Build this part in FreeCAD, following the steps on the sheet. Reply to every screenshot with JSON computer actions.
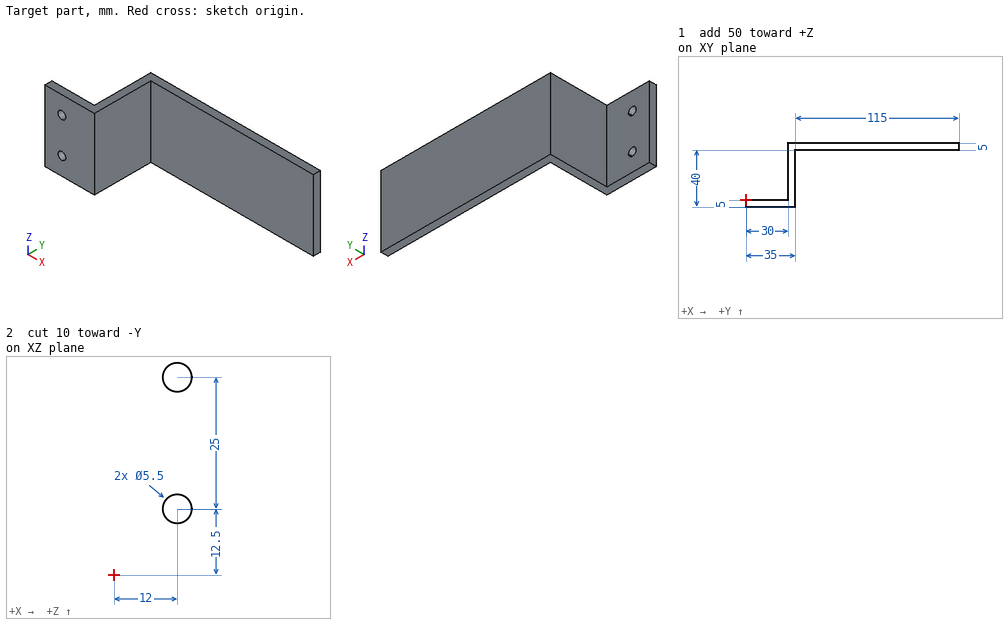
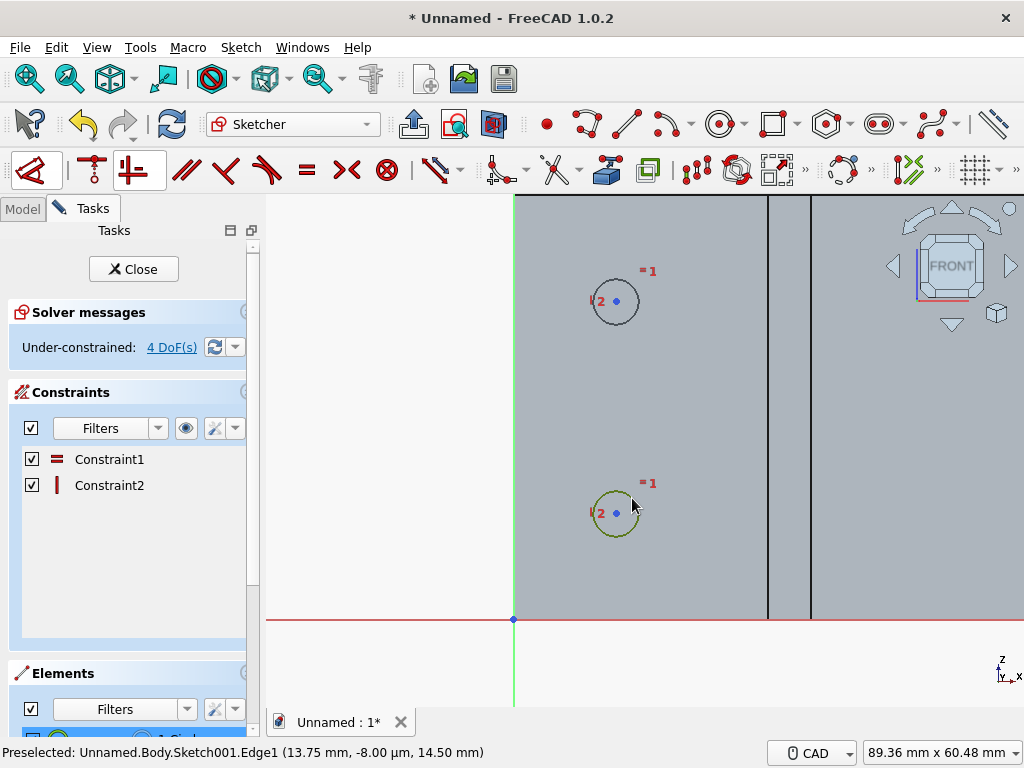
{"action": "left_click", "coordinate": [56, 170]}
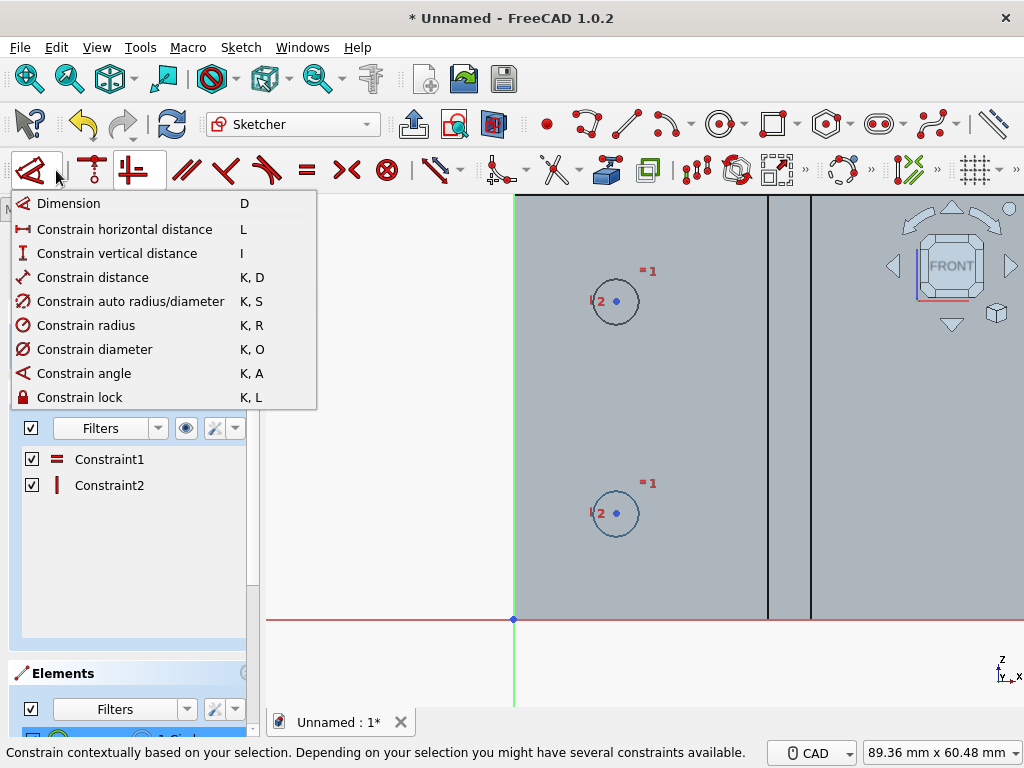
{"action": "left_click", "coordinate": [164, 349]}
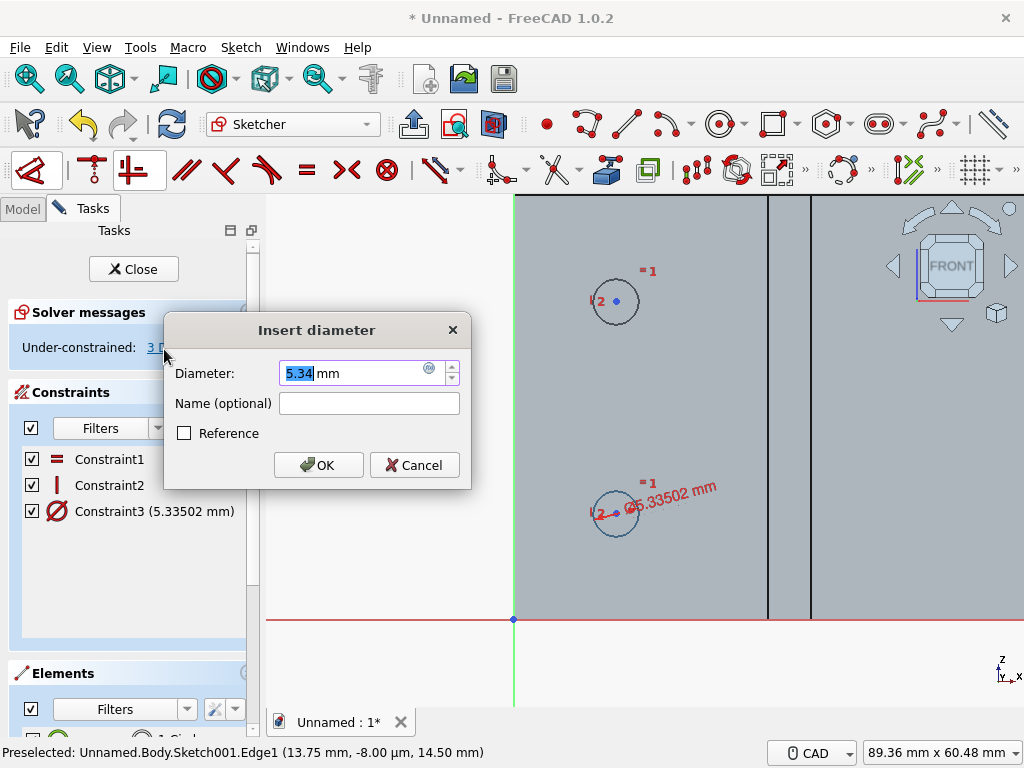
{"action": "type", "text": "5.5"}
{"action": "key", "text": "Return"}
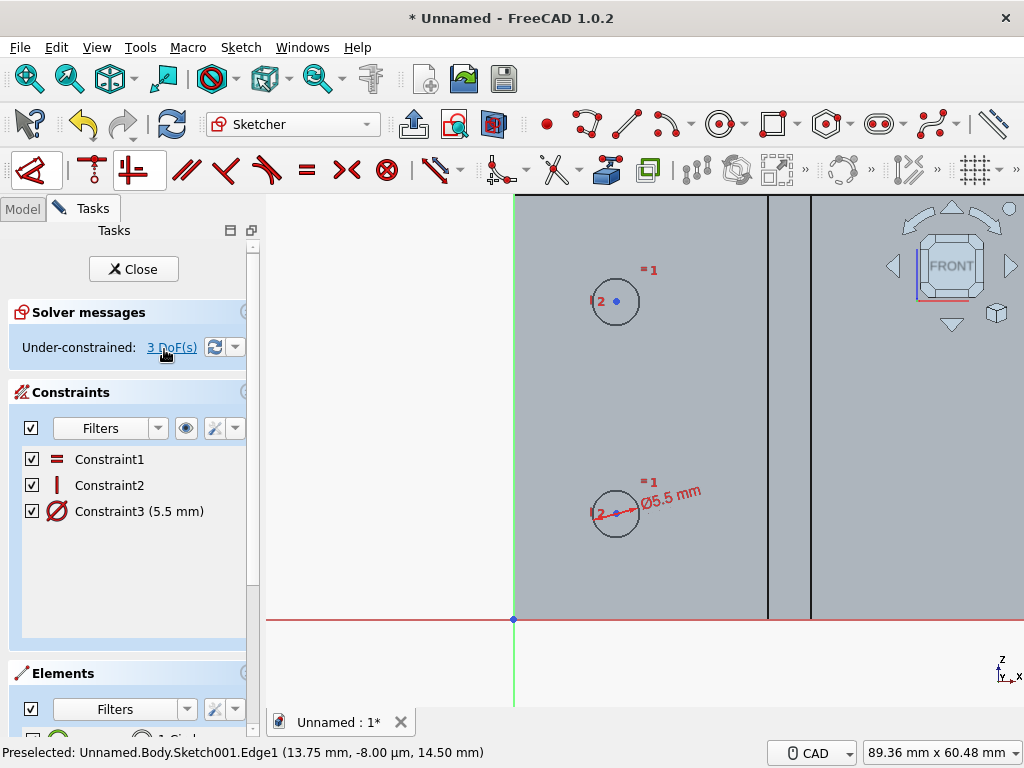
{"action": "left_click", "coordinate": [616, 514]}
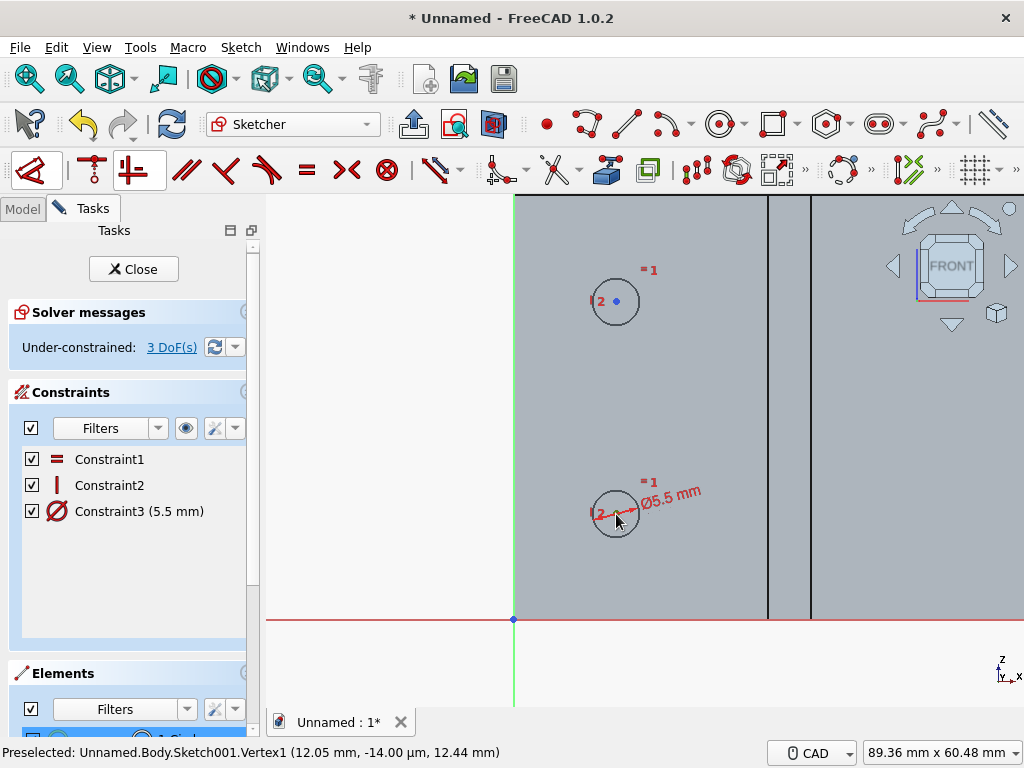
{"action": "key", "text": "l"}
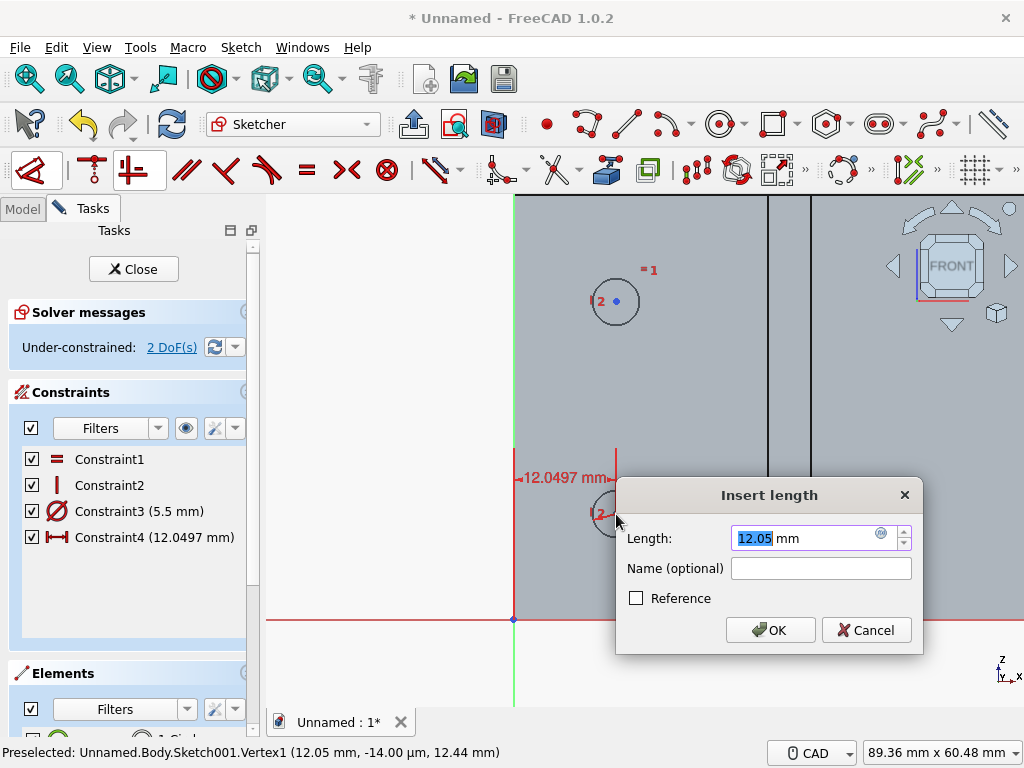
{"action": "type", "text": "12"}
{"action": "key", "text": "Return"}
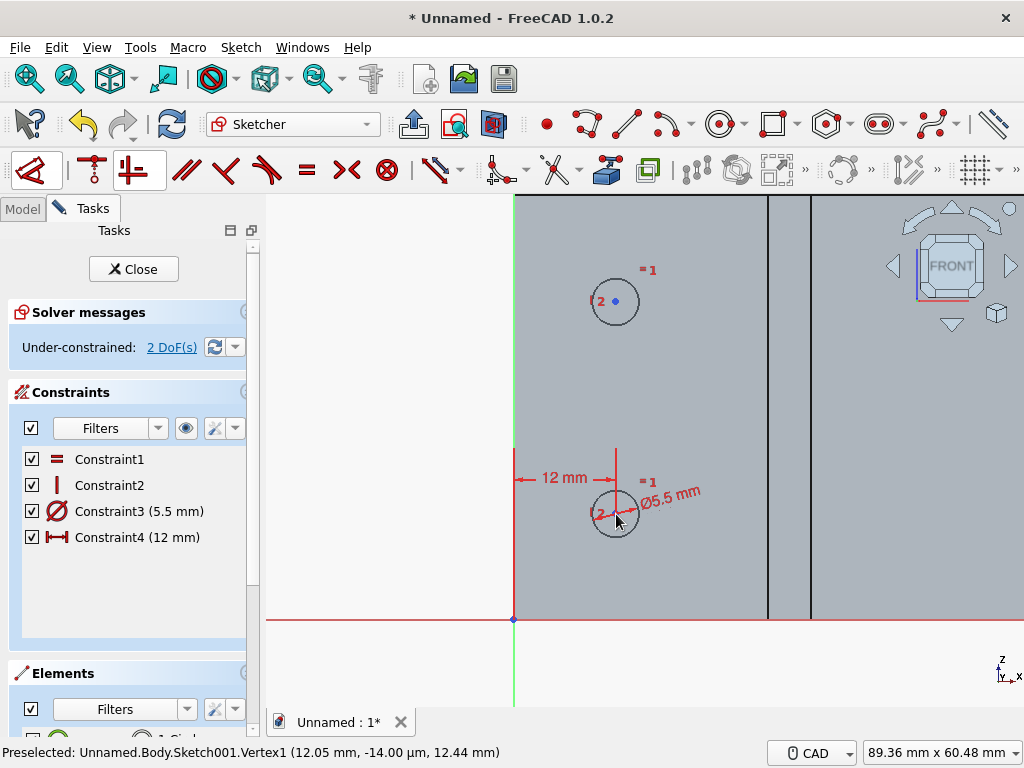
{"action": "left_click", "coordinate": [616, 514]}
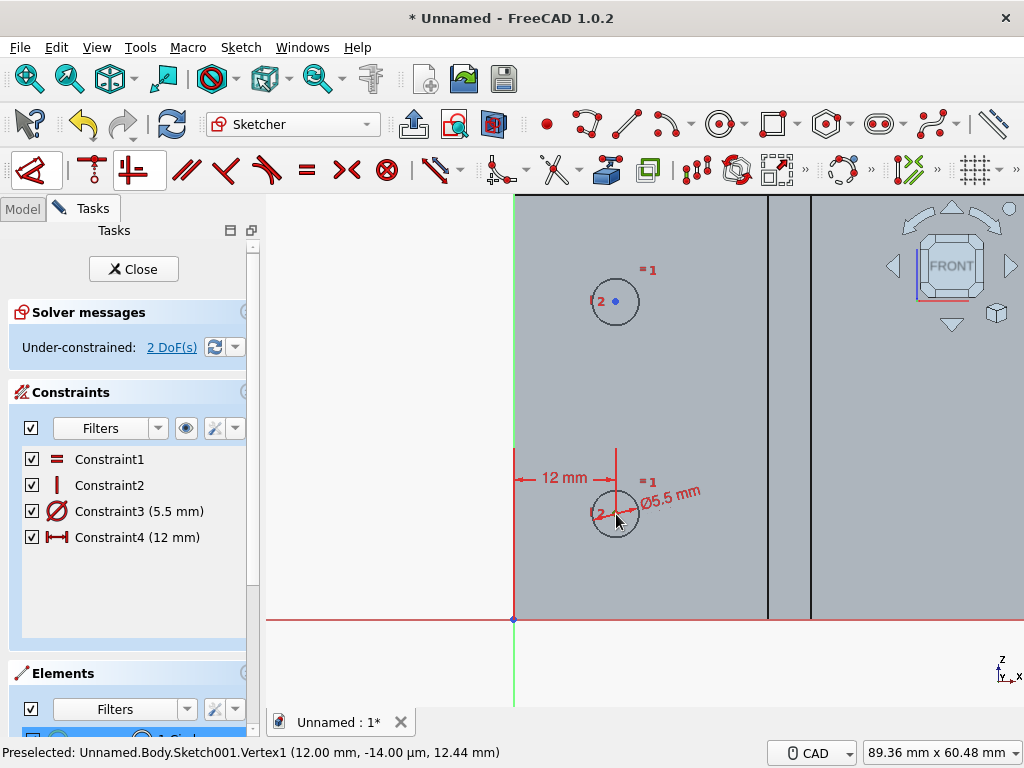
{"action": "left_click", "coordinate": [616, 302]}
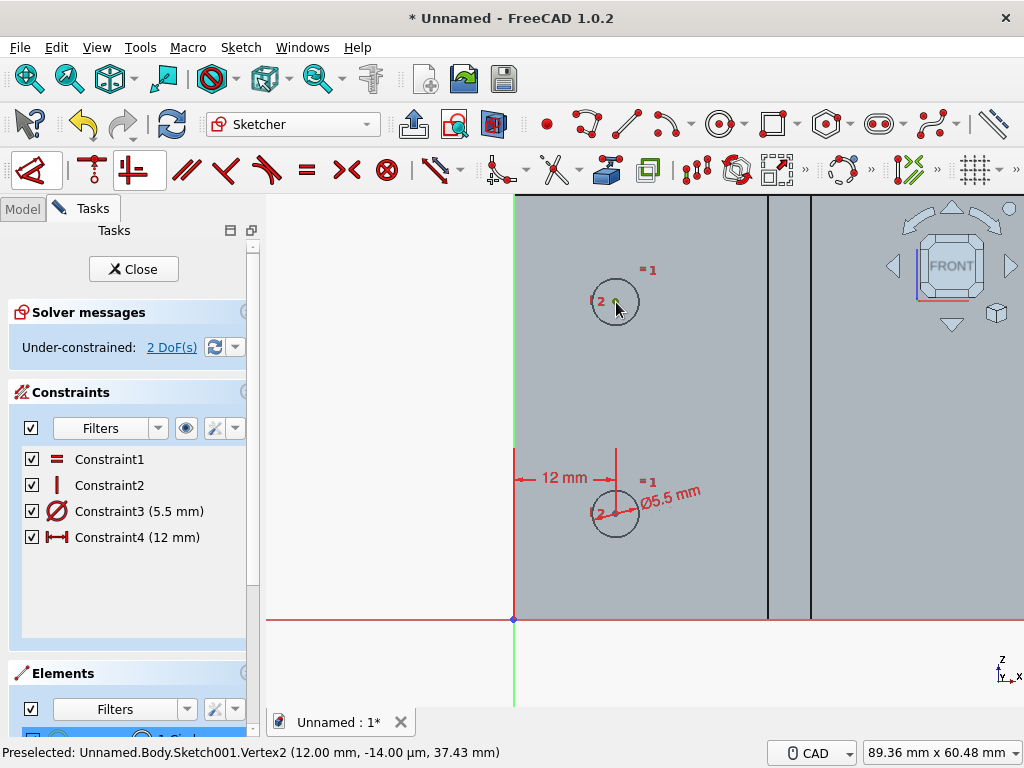
{"action": "key", "text": "i"}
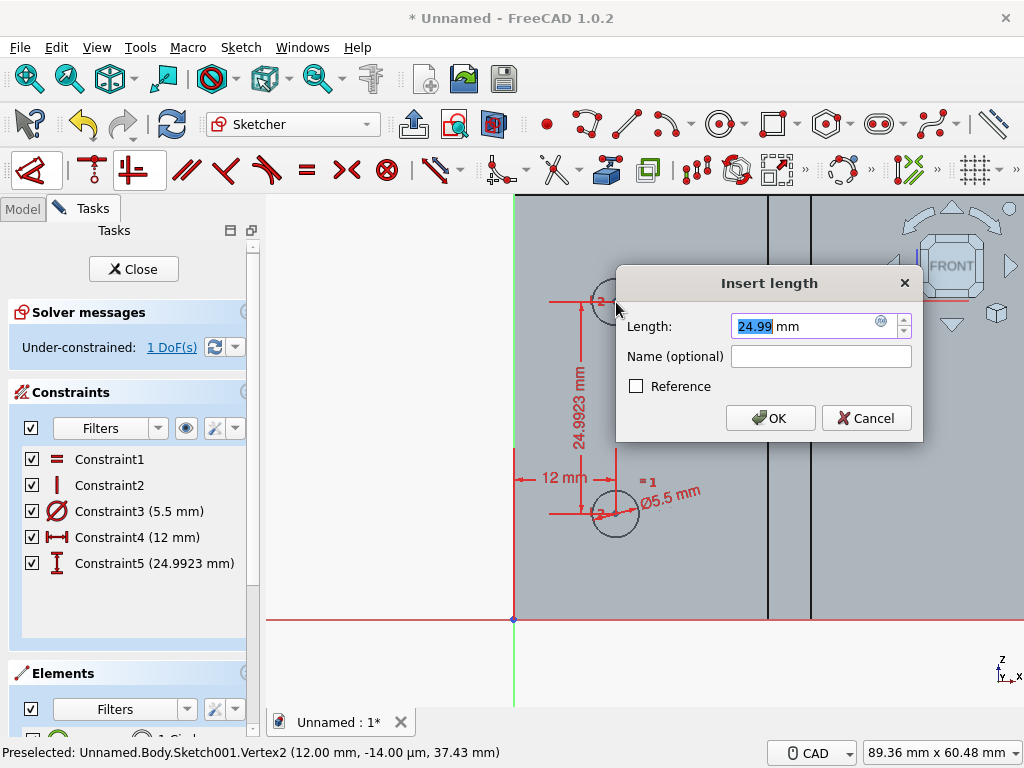
{"action": "type", "text": "25"}
{"action": "key", "text": "Return"}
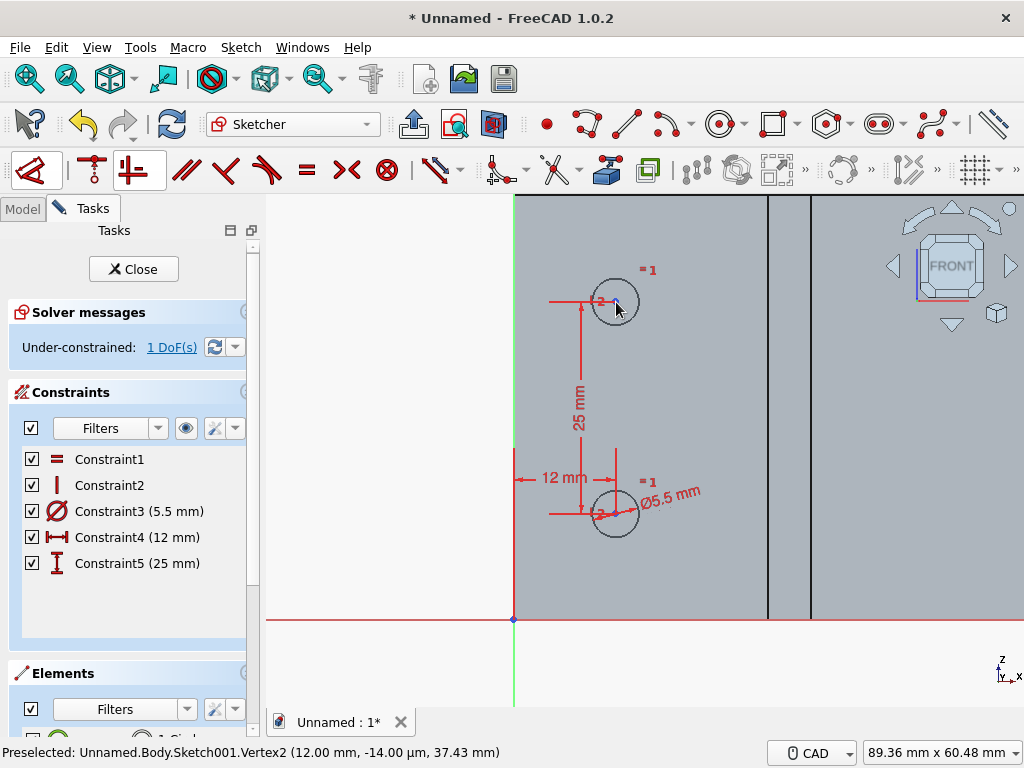
{"action": "left_click", "coordinate": [616, 514]}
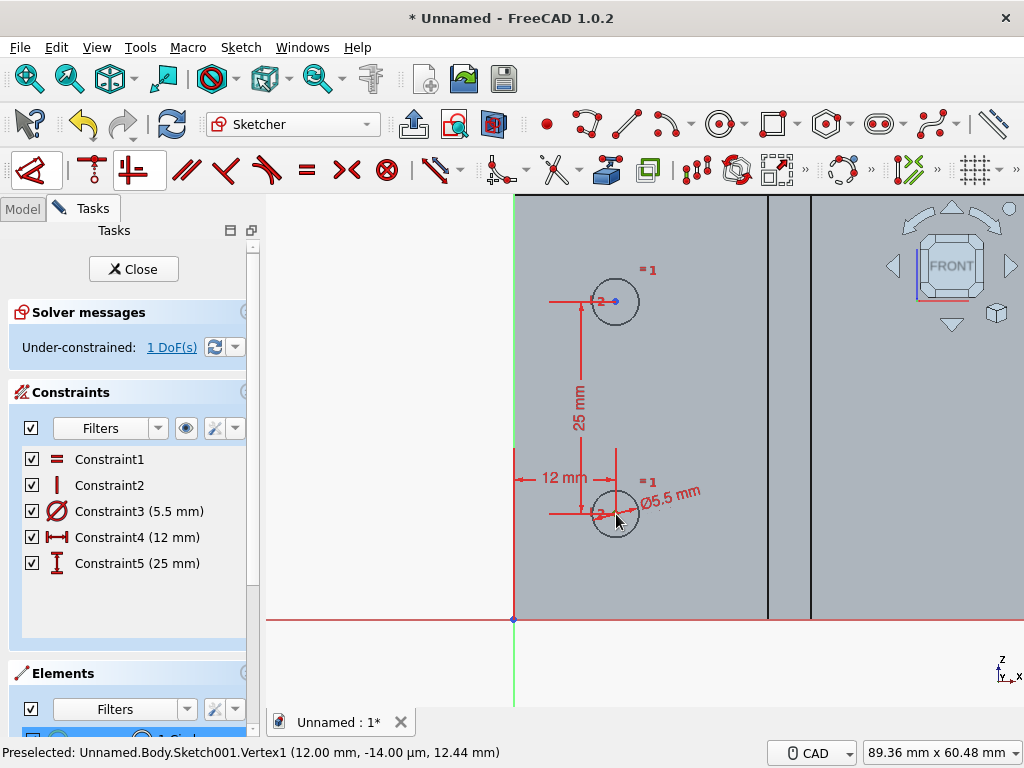
{"action": "key", "text": "i"}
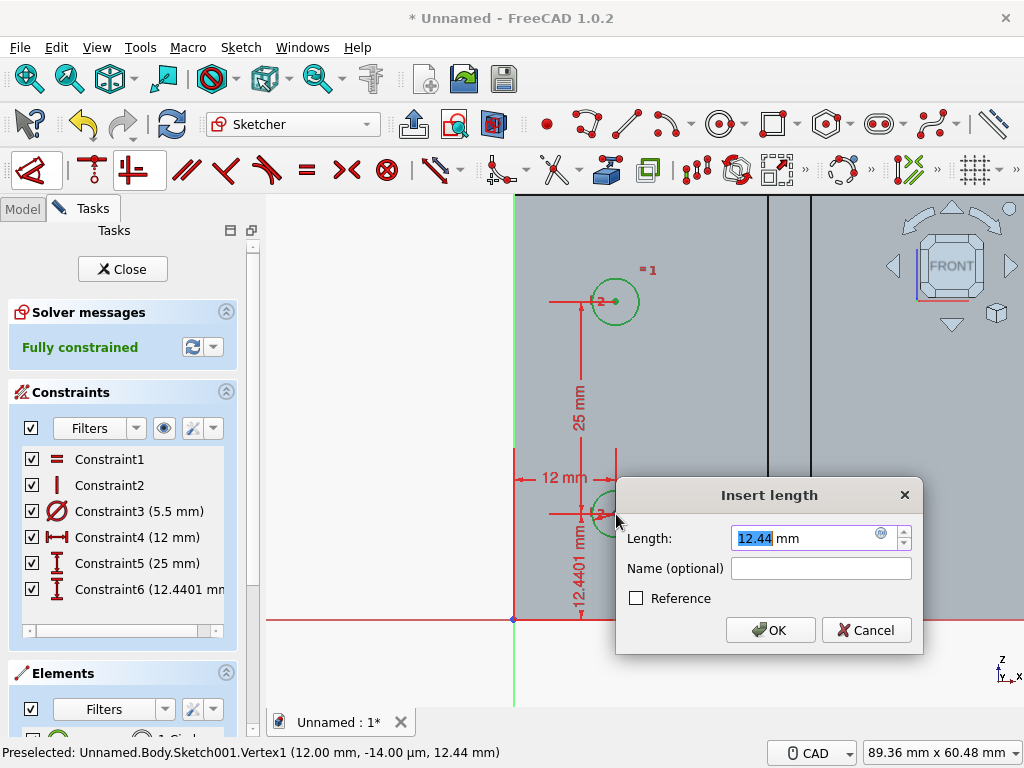
{"action": "type", "text": "12.5"}
{"action": "key", "text": "Return"}